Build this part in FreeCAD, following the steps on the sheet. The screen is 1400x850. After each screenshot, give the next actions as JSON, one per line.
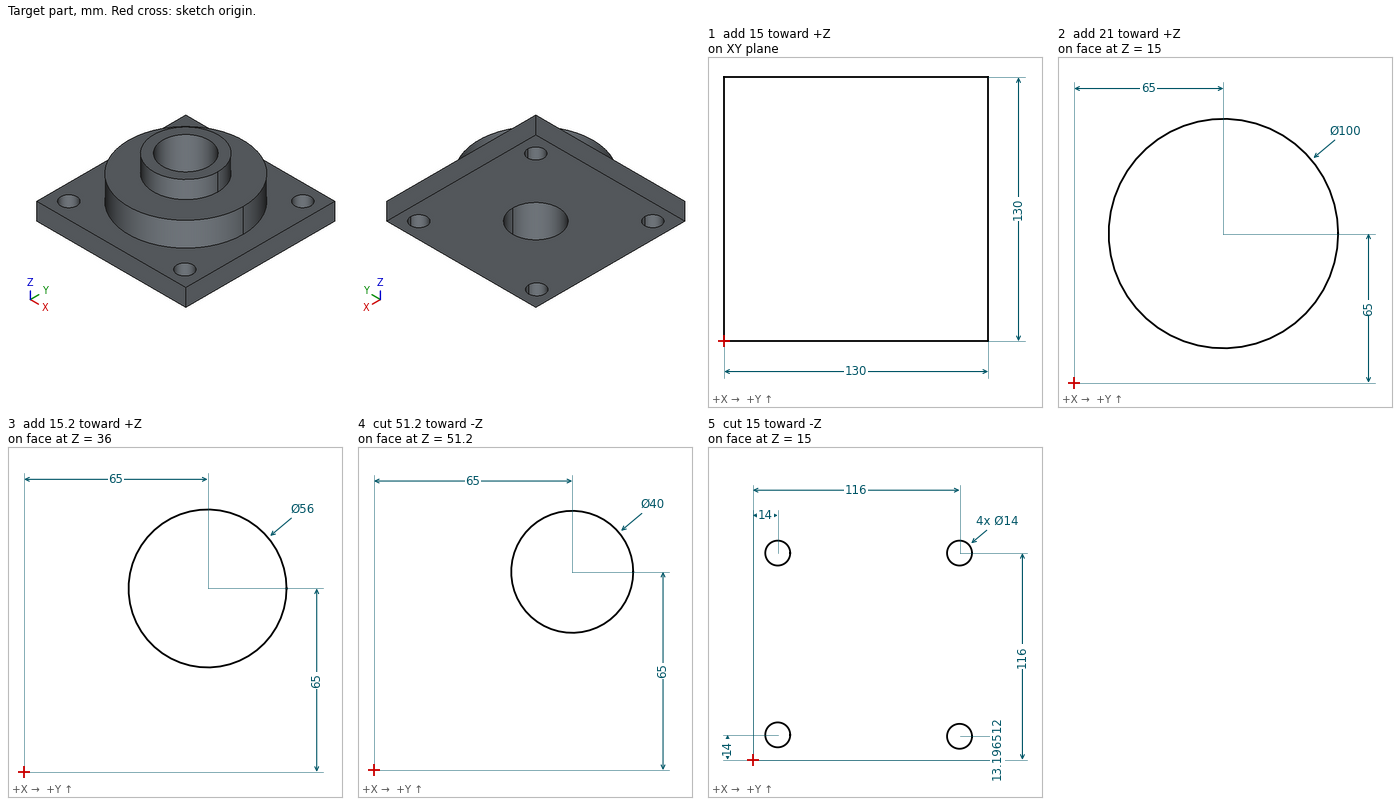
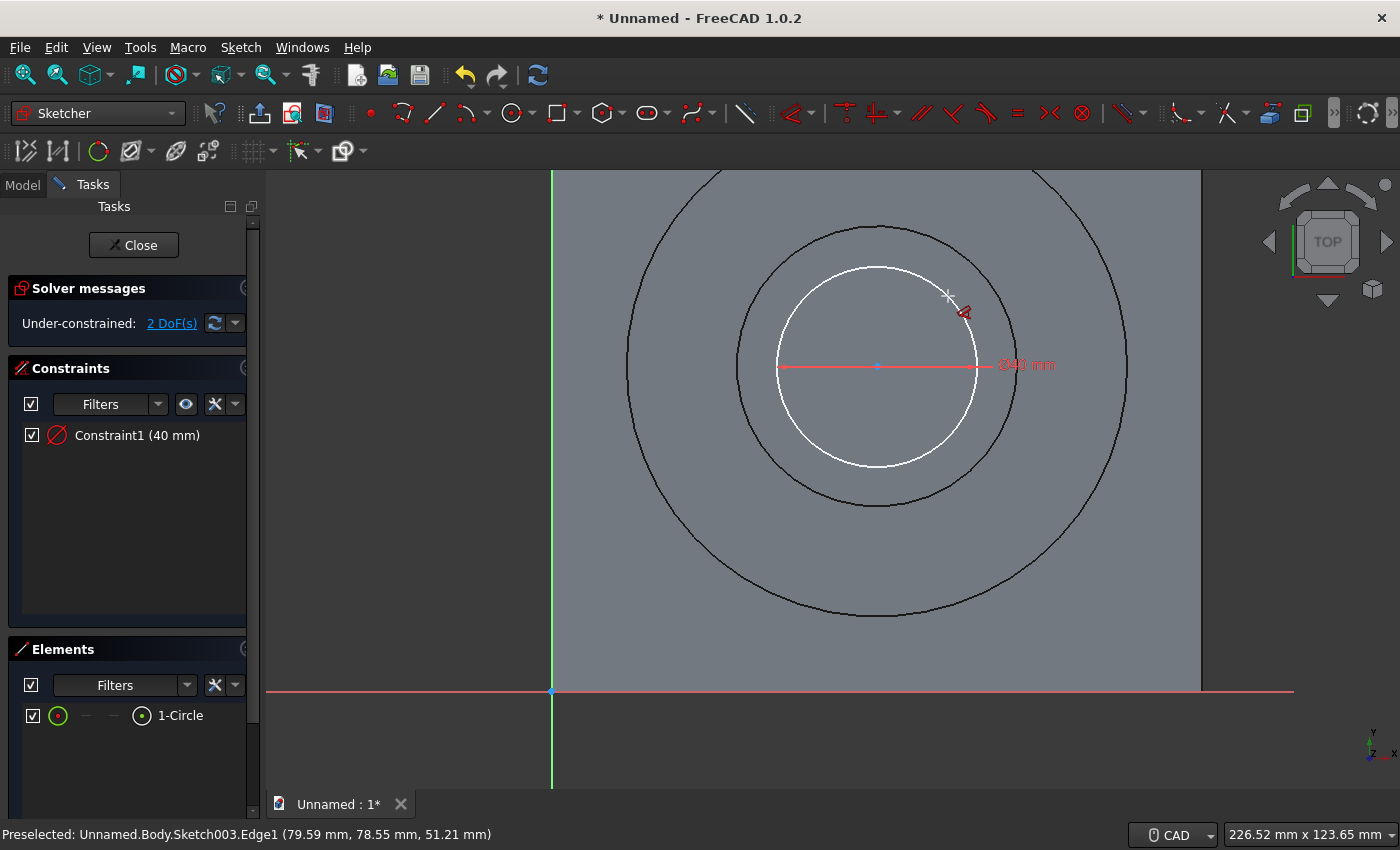
{"action": "left_click", "coordinate": [877, 367]}
{"action": "left_click", "coordinate": [714, 726]}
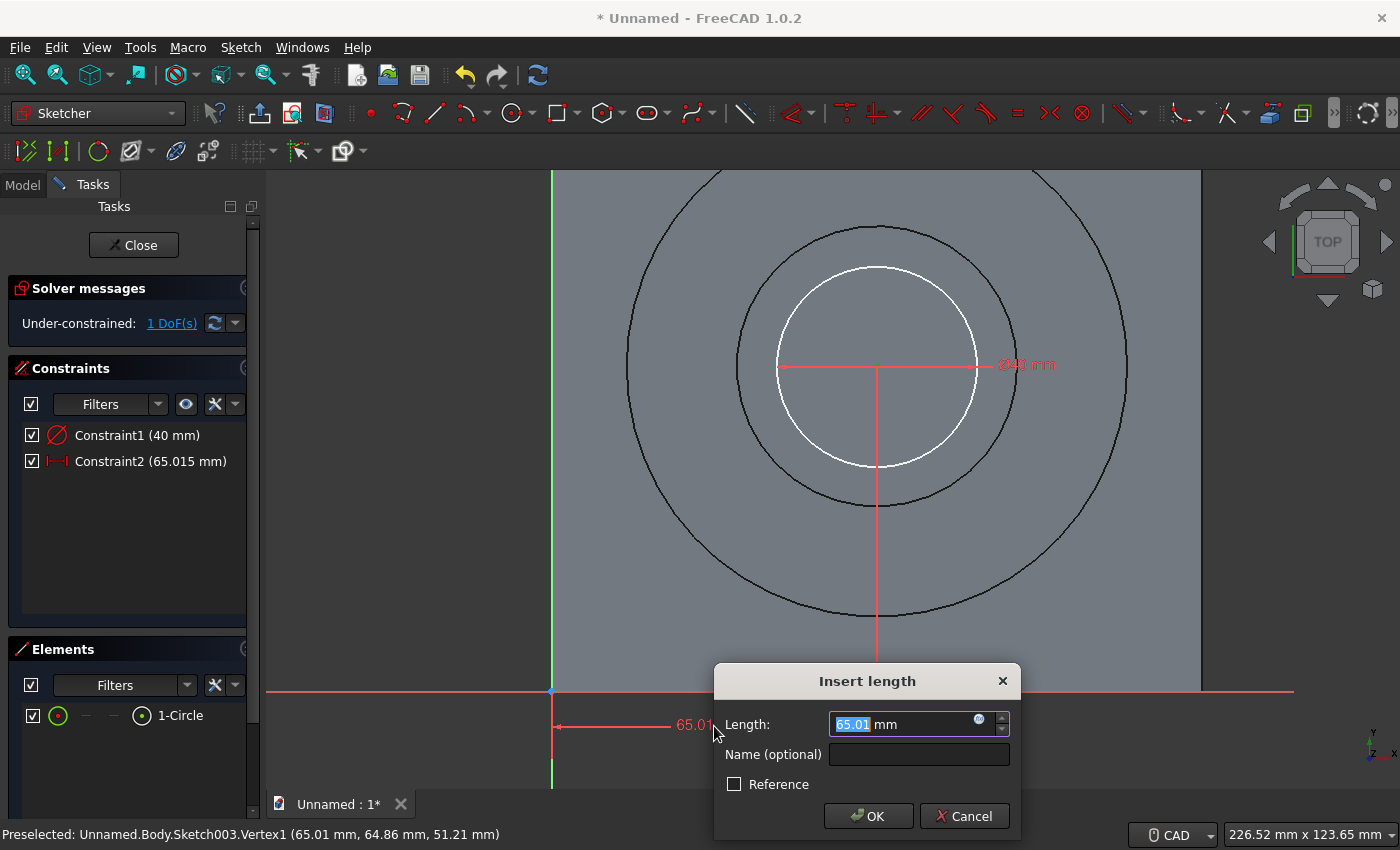
{"action": "type", "text": "65"}
{"action": "key", "text": "Return"}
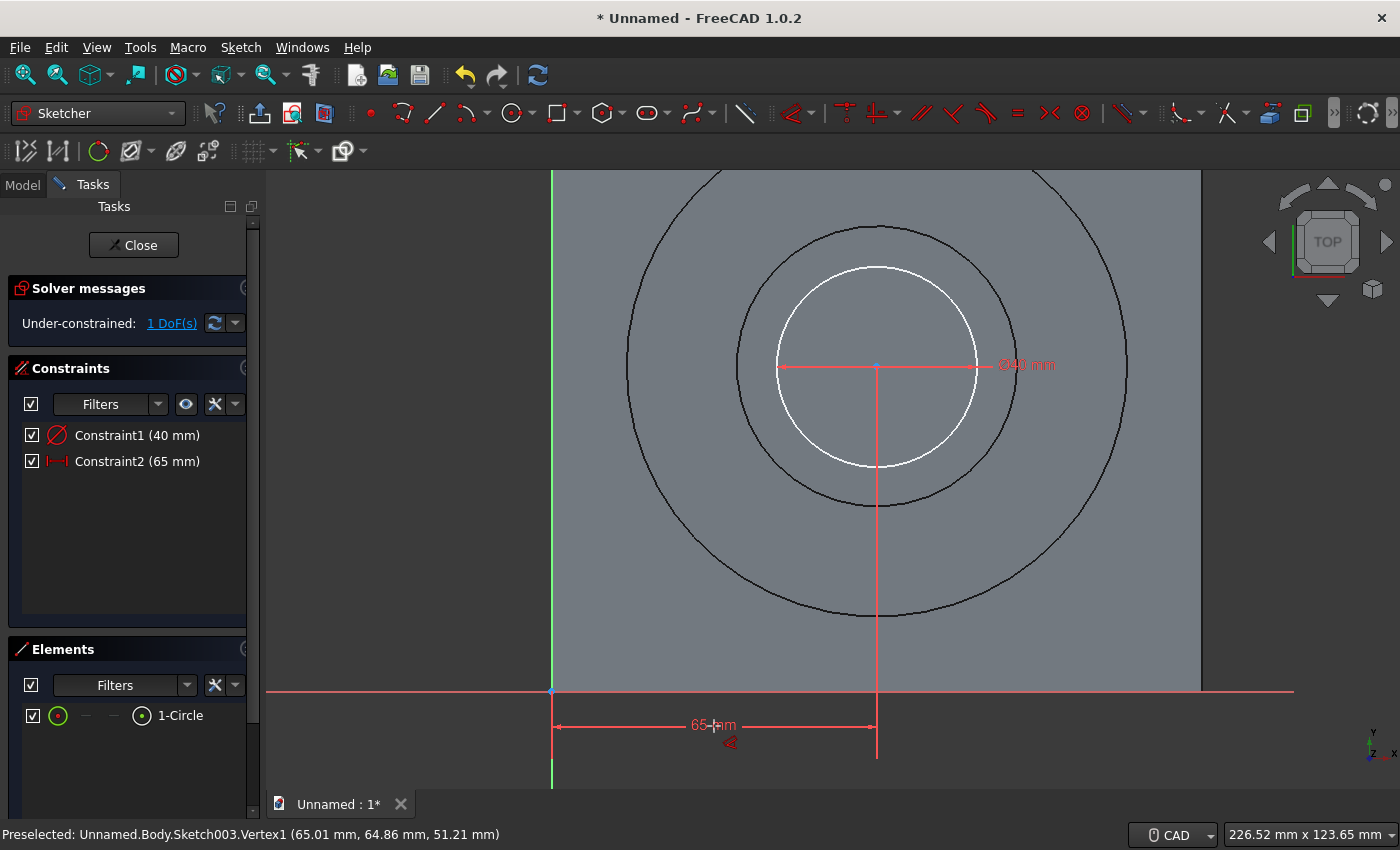
{"action": "left_click", "coordinate": [877, 367]}
{"action": "left_click", "coordinate": [518, 529]}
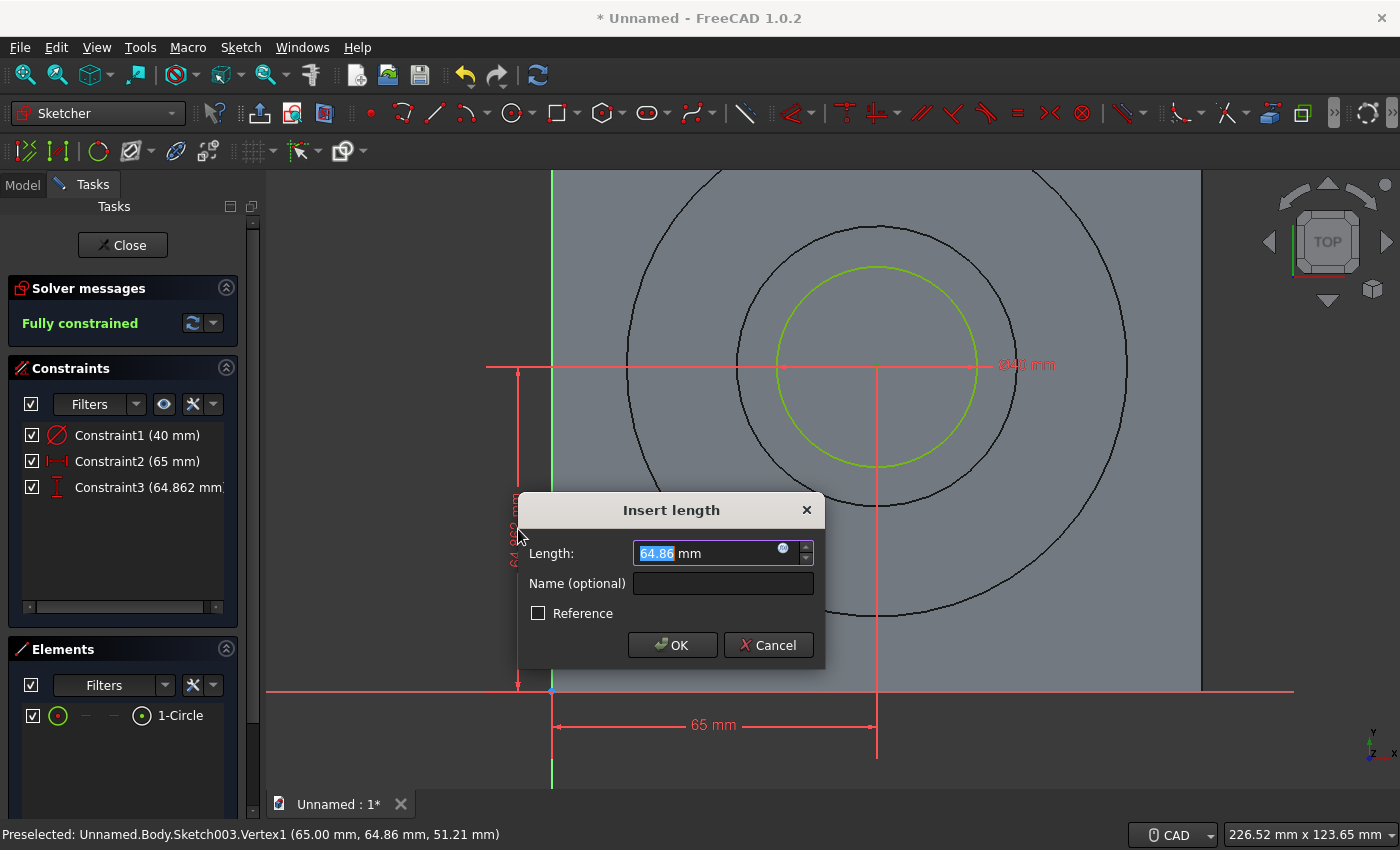
{"action": "type", "text": "65"}
{"action": "key", "text": "Return"}
{"action": "key", "text": "Escape"}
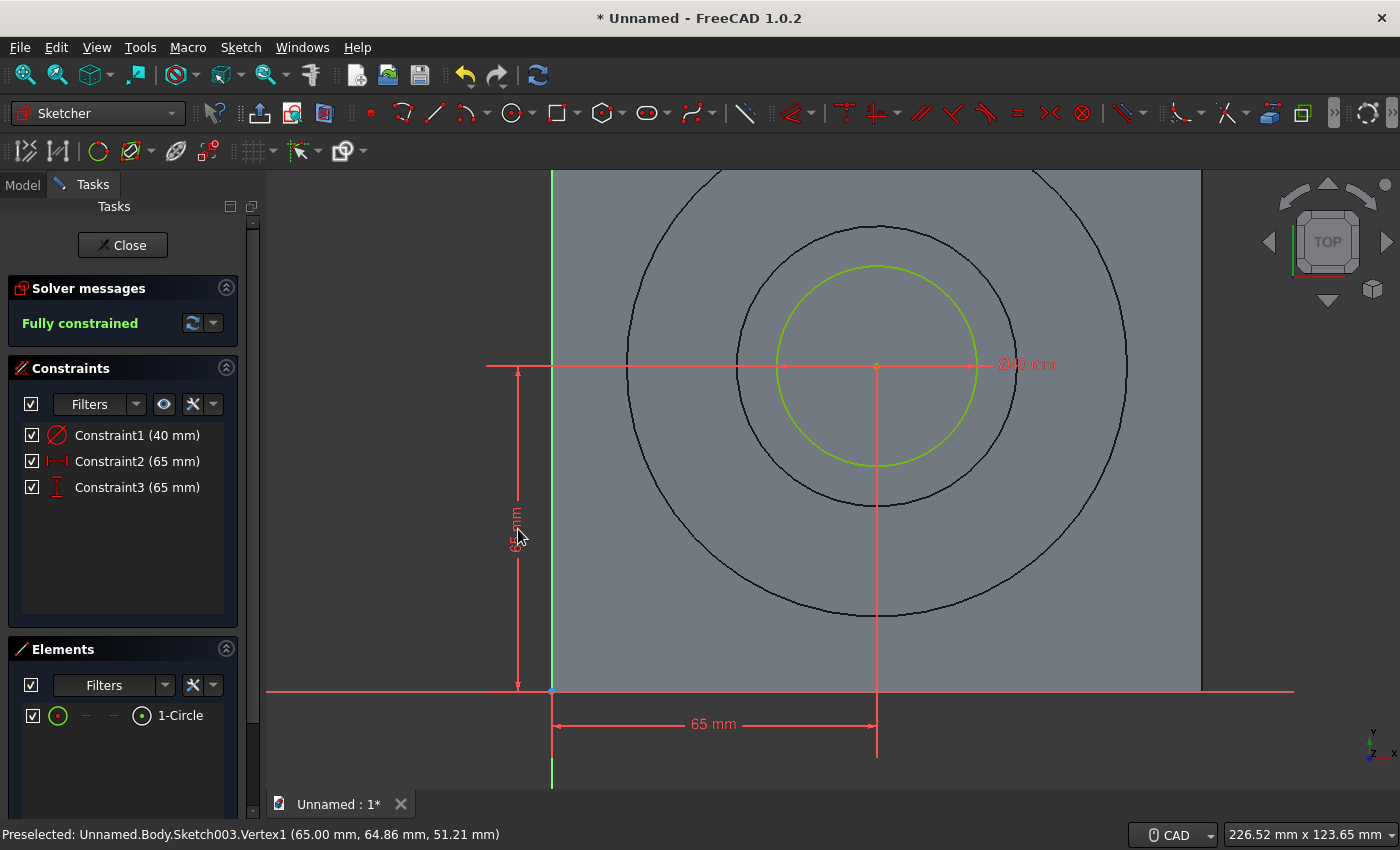
{"action": "left_click", "coordinate": [123, 245]}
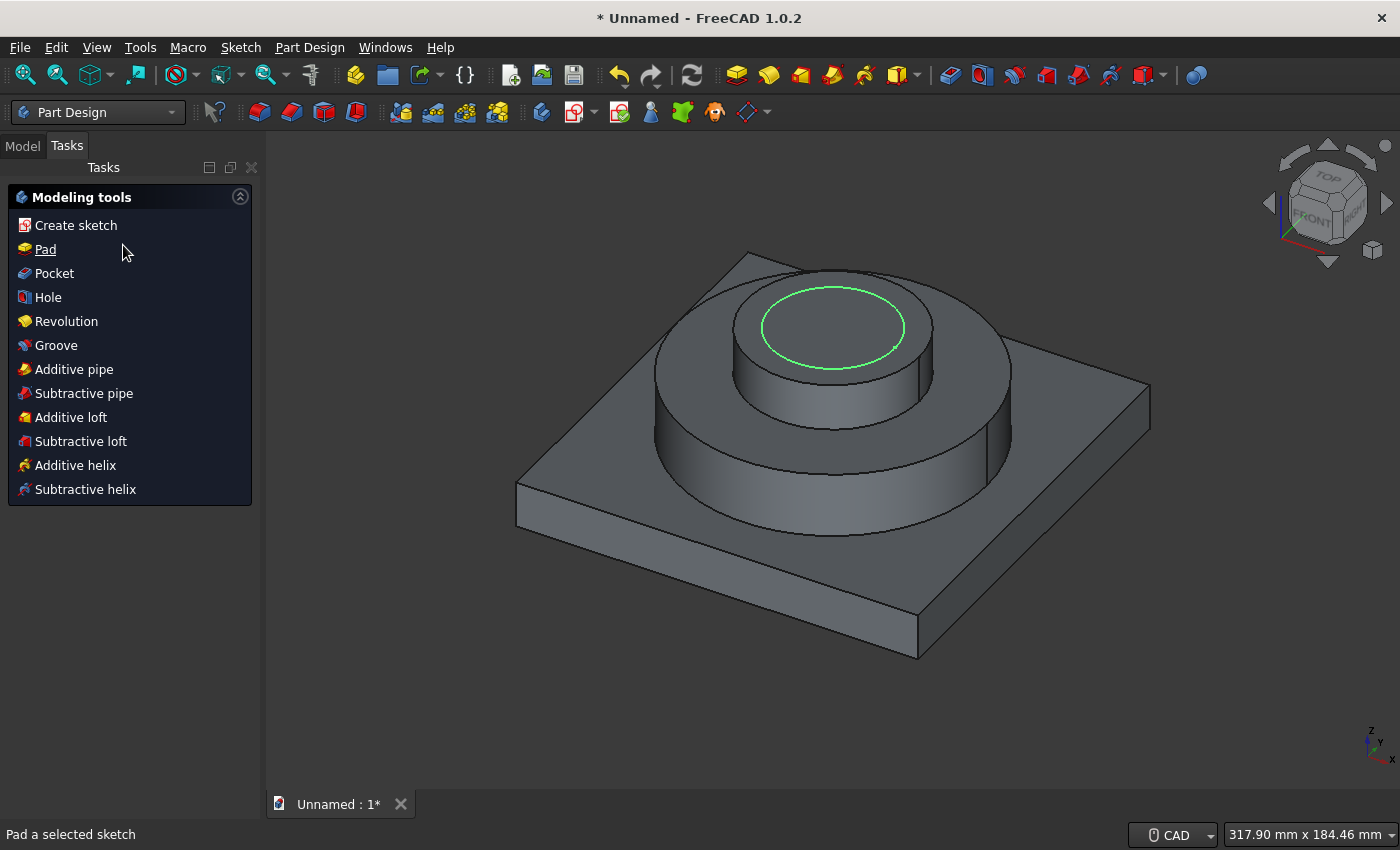
{"action": "left_click", "coordinate": [952, 76]}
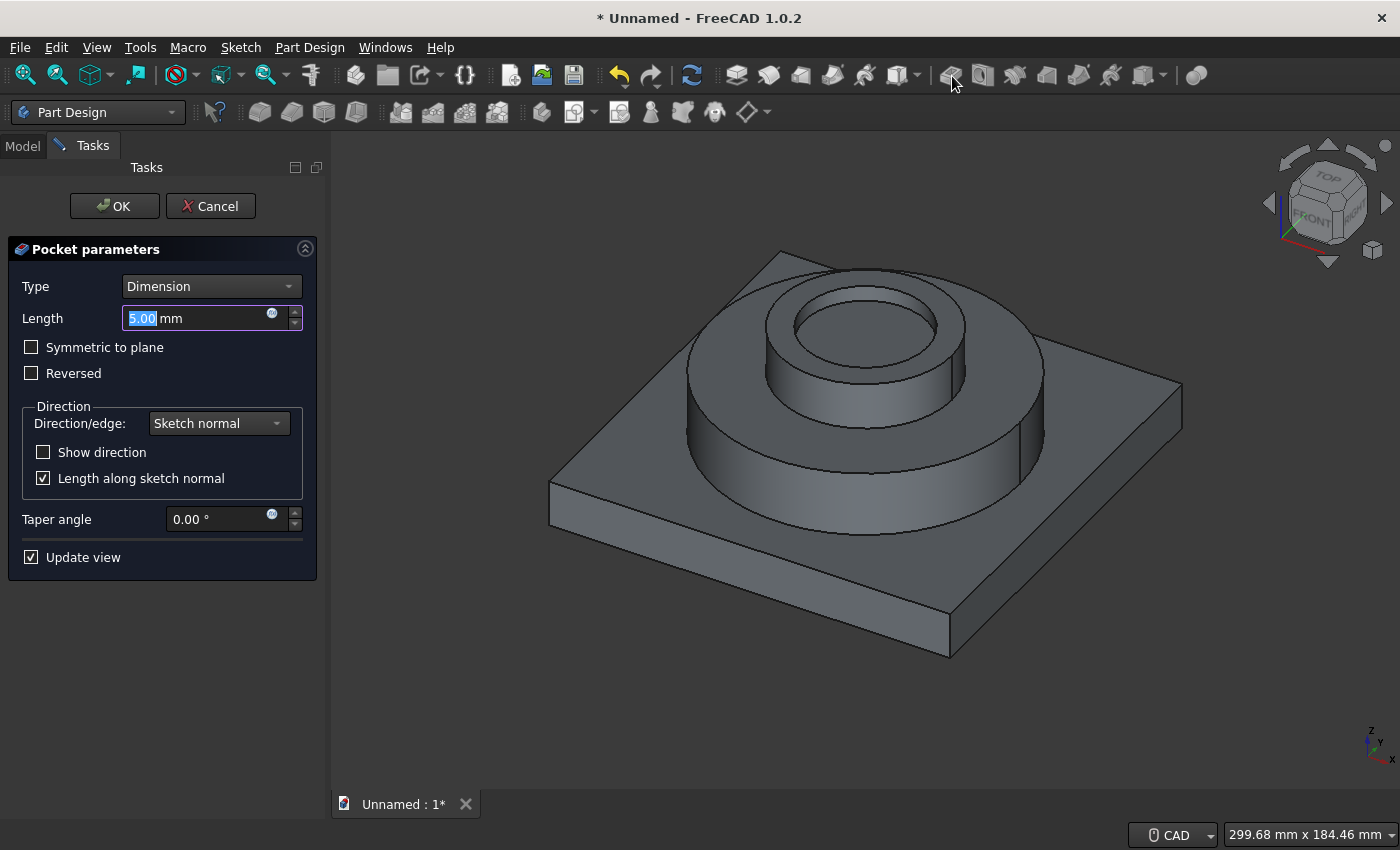
{"action": "type", "text": "51.2"}
{"action": "key", "text": "Tab"}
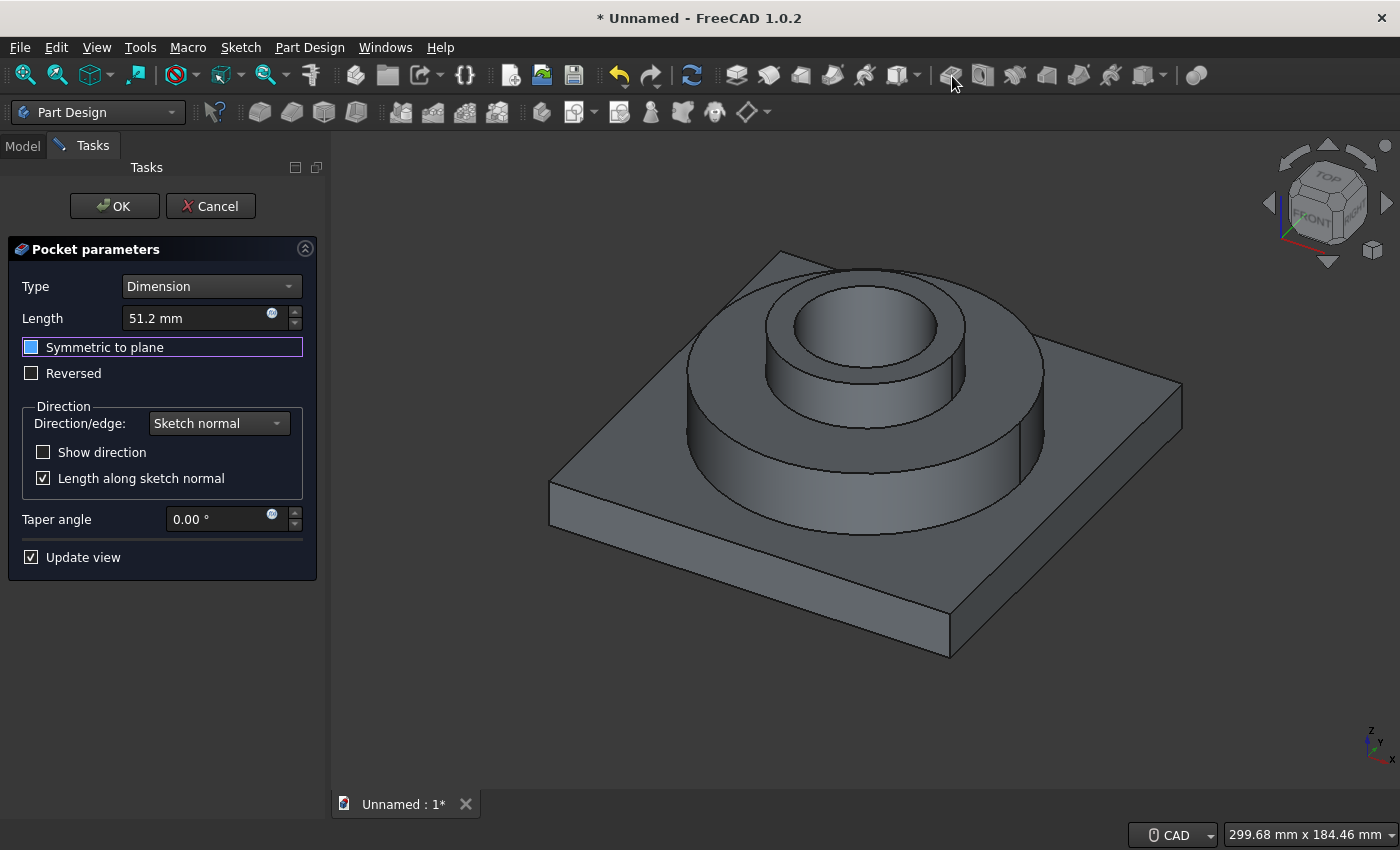
{"action": "left_click", "coordinate": [115, 206]}